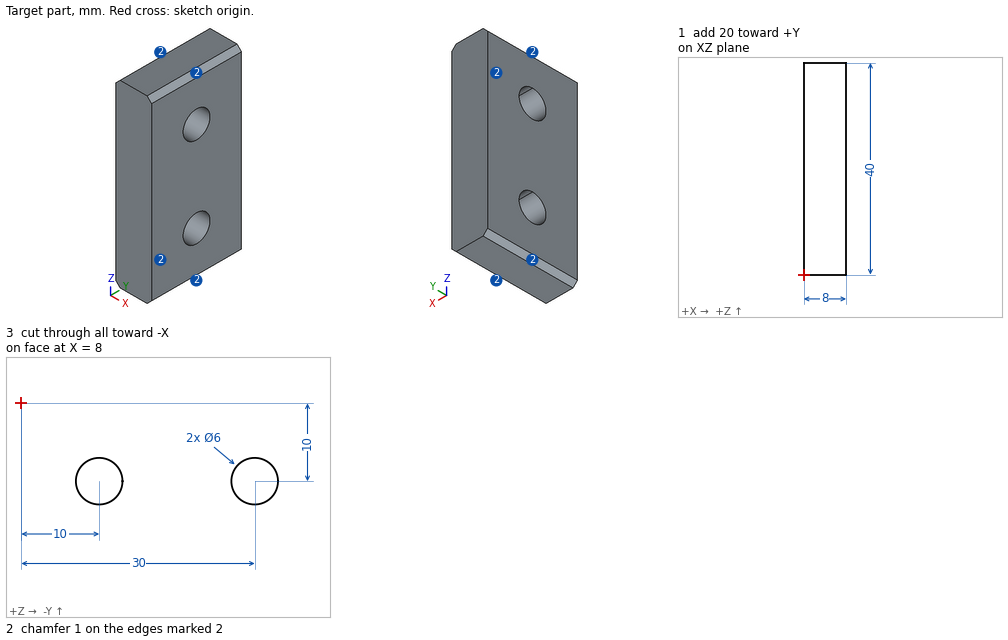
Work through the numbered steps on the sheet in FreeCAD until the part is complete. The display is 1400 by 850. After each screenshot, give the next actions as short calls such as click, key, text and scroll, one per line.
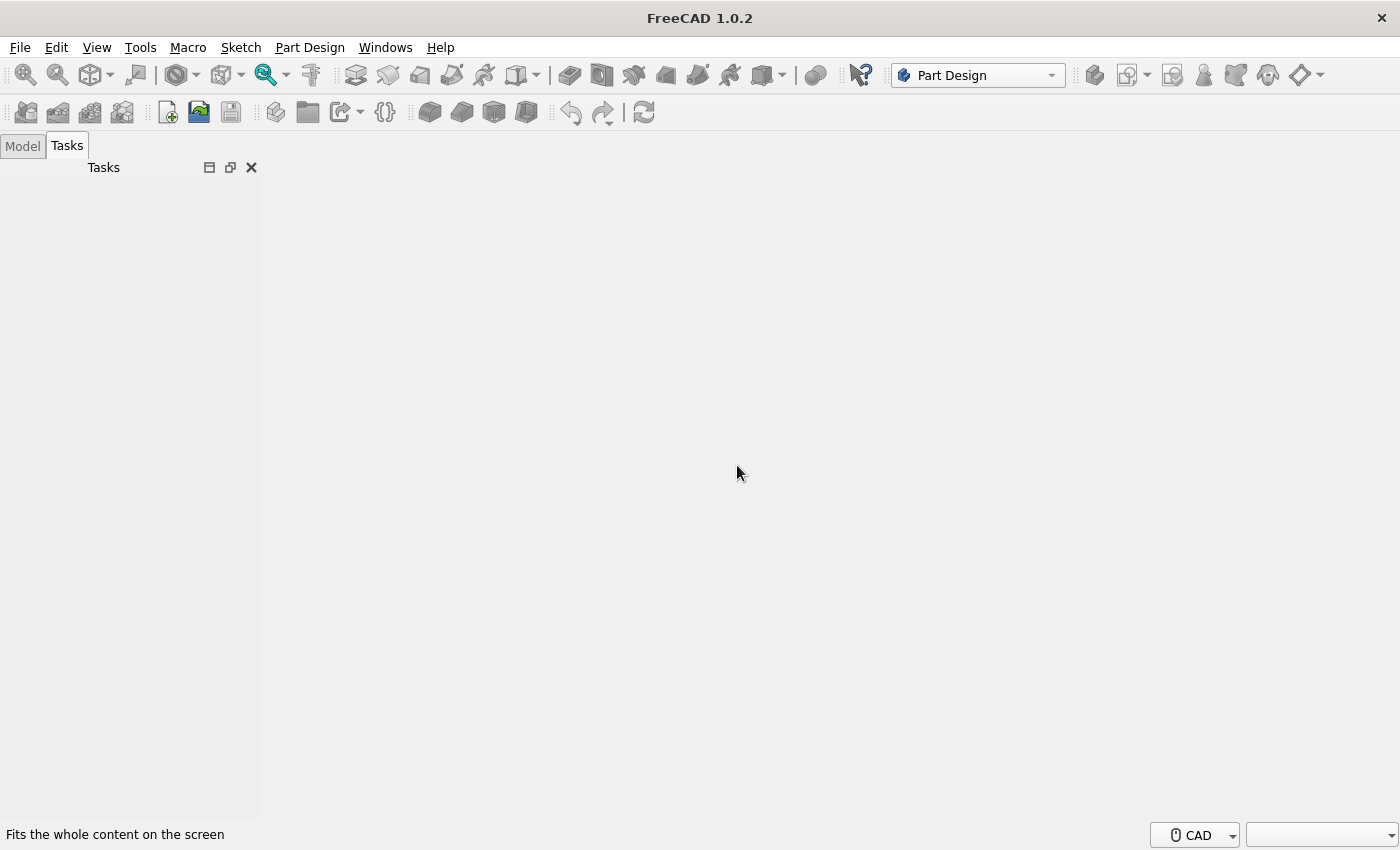
click(168, 112)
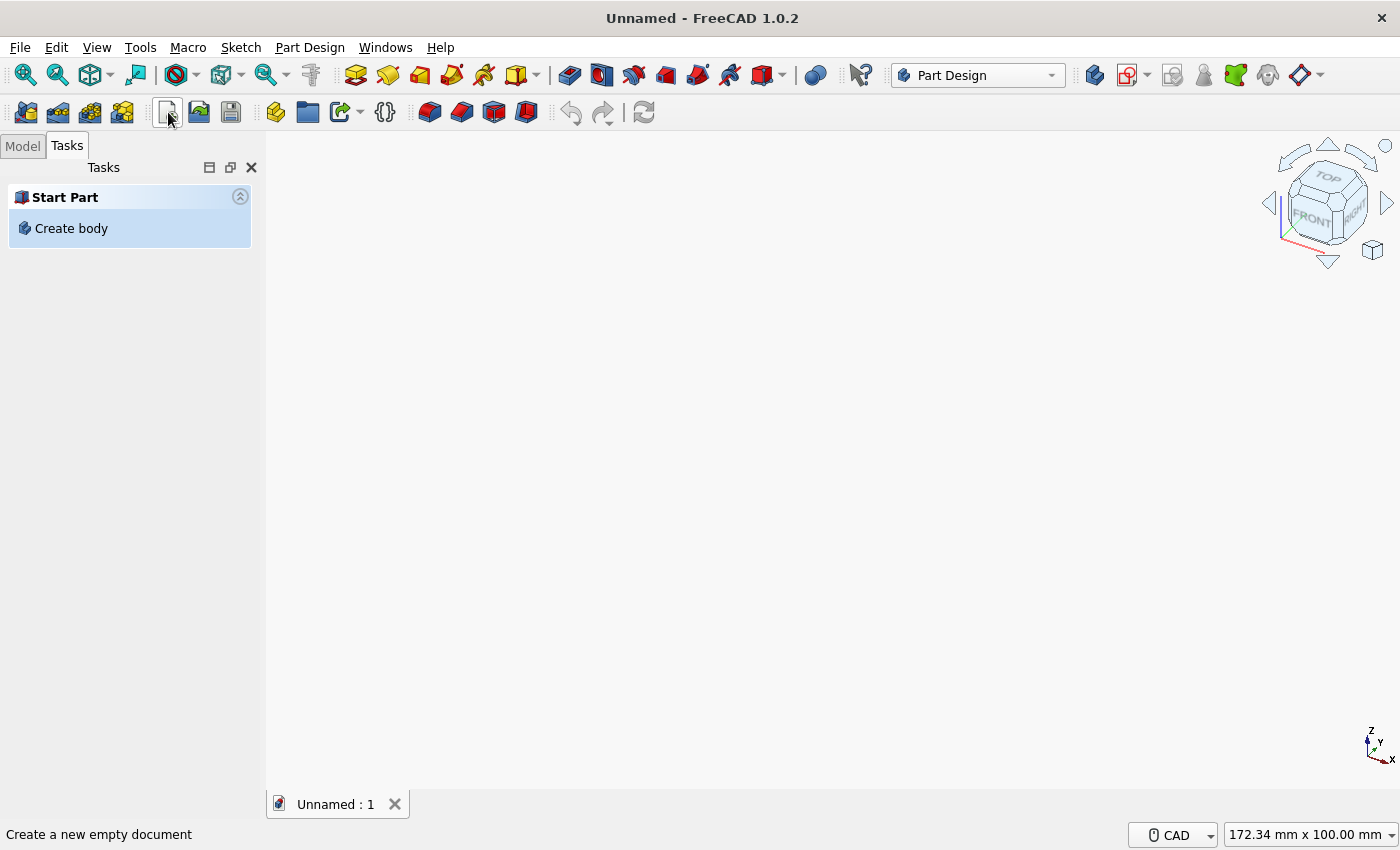
click(1128, 76)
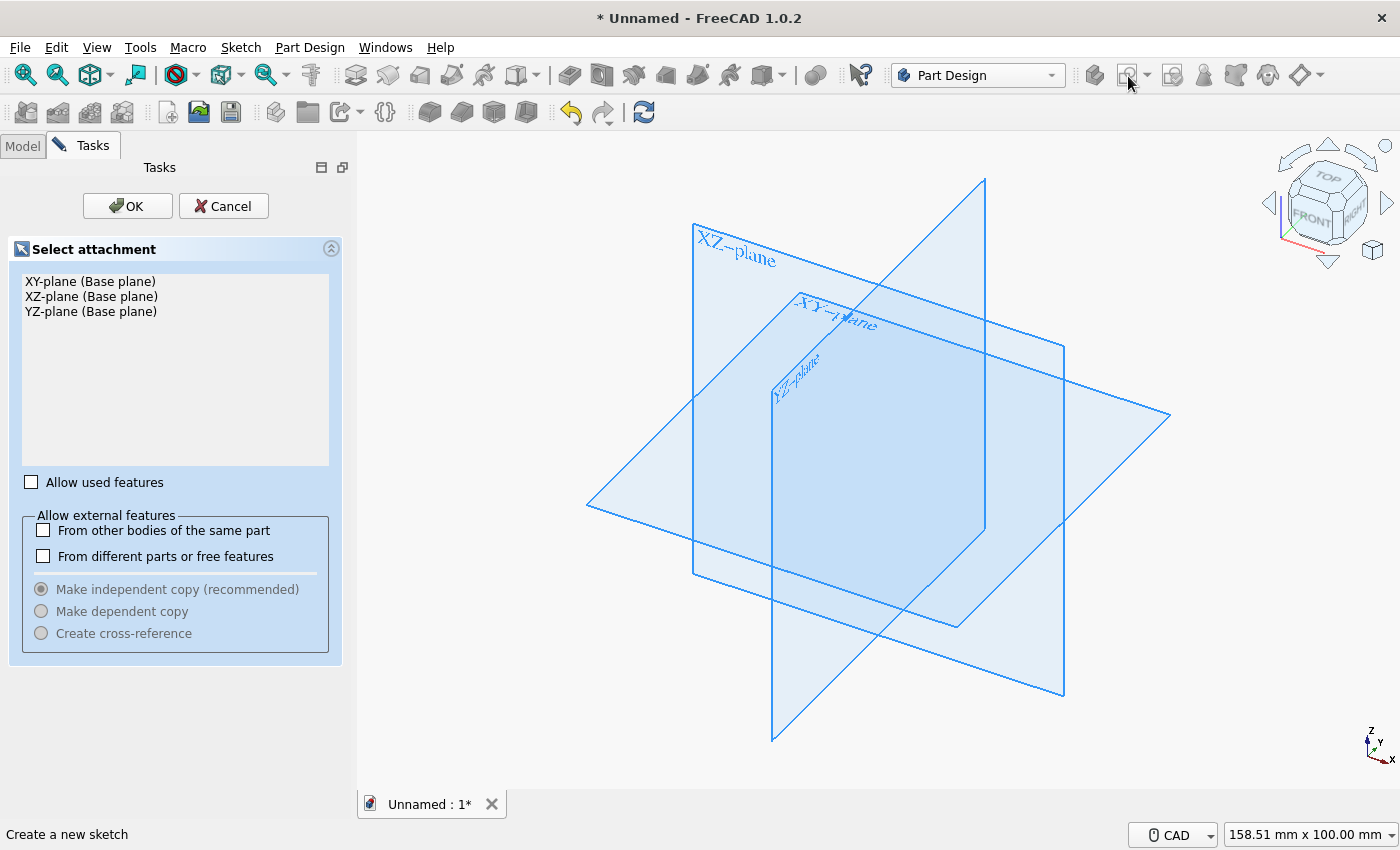
click(82, 296)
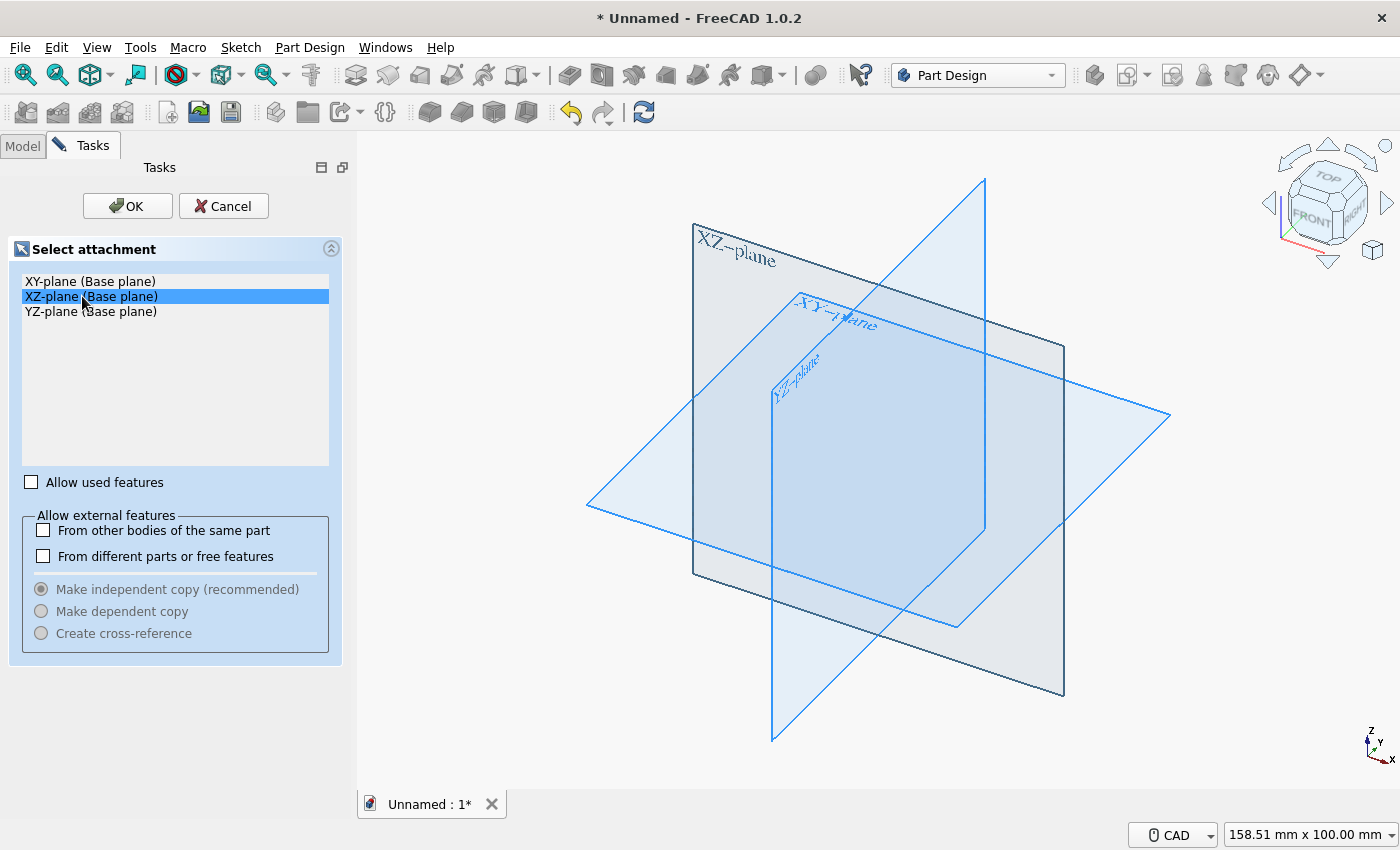
click(128, 206)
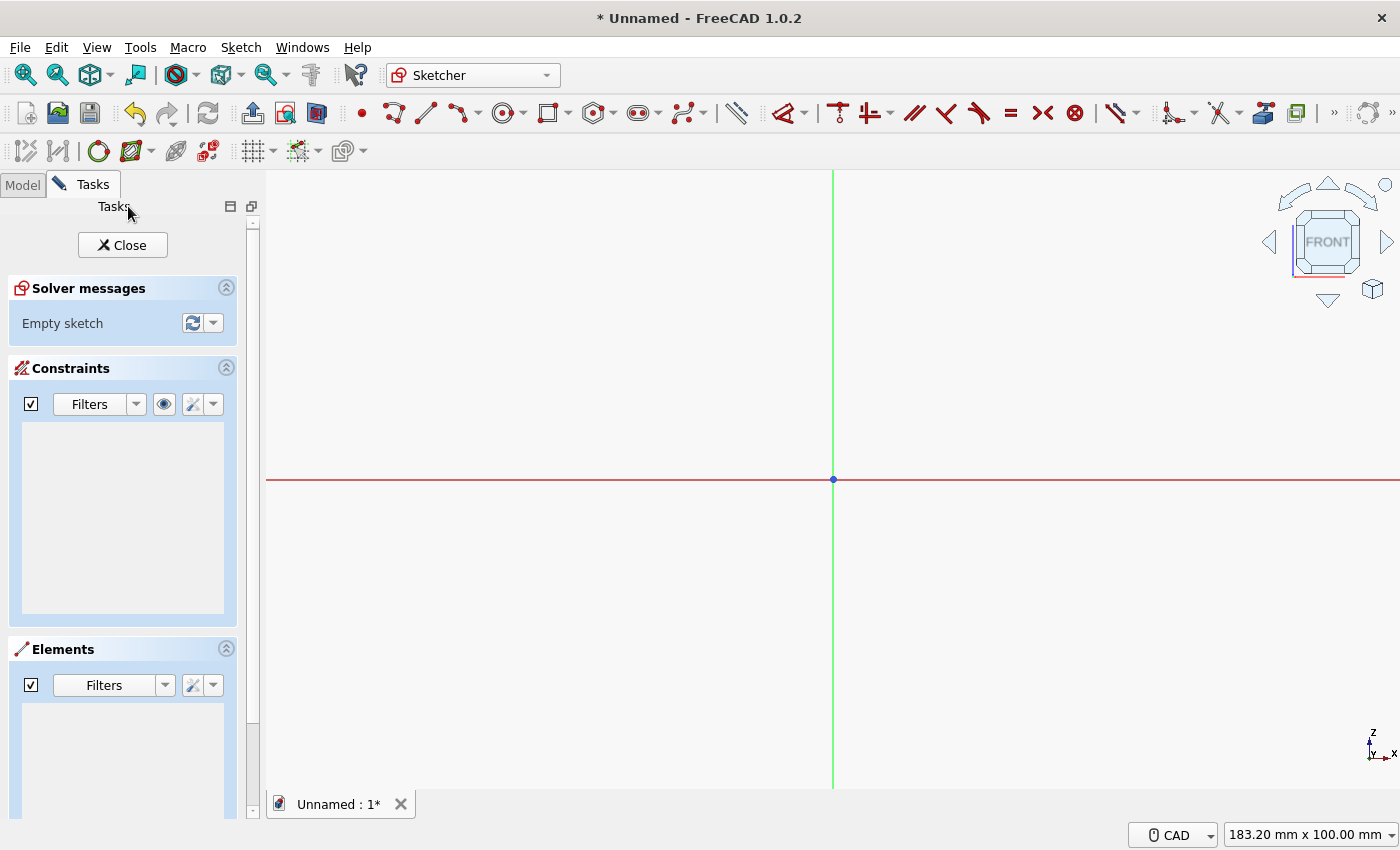
scroll(1047, 198, up, 2)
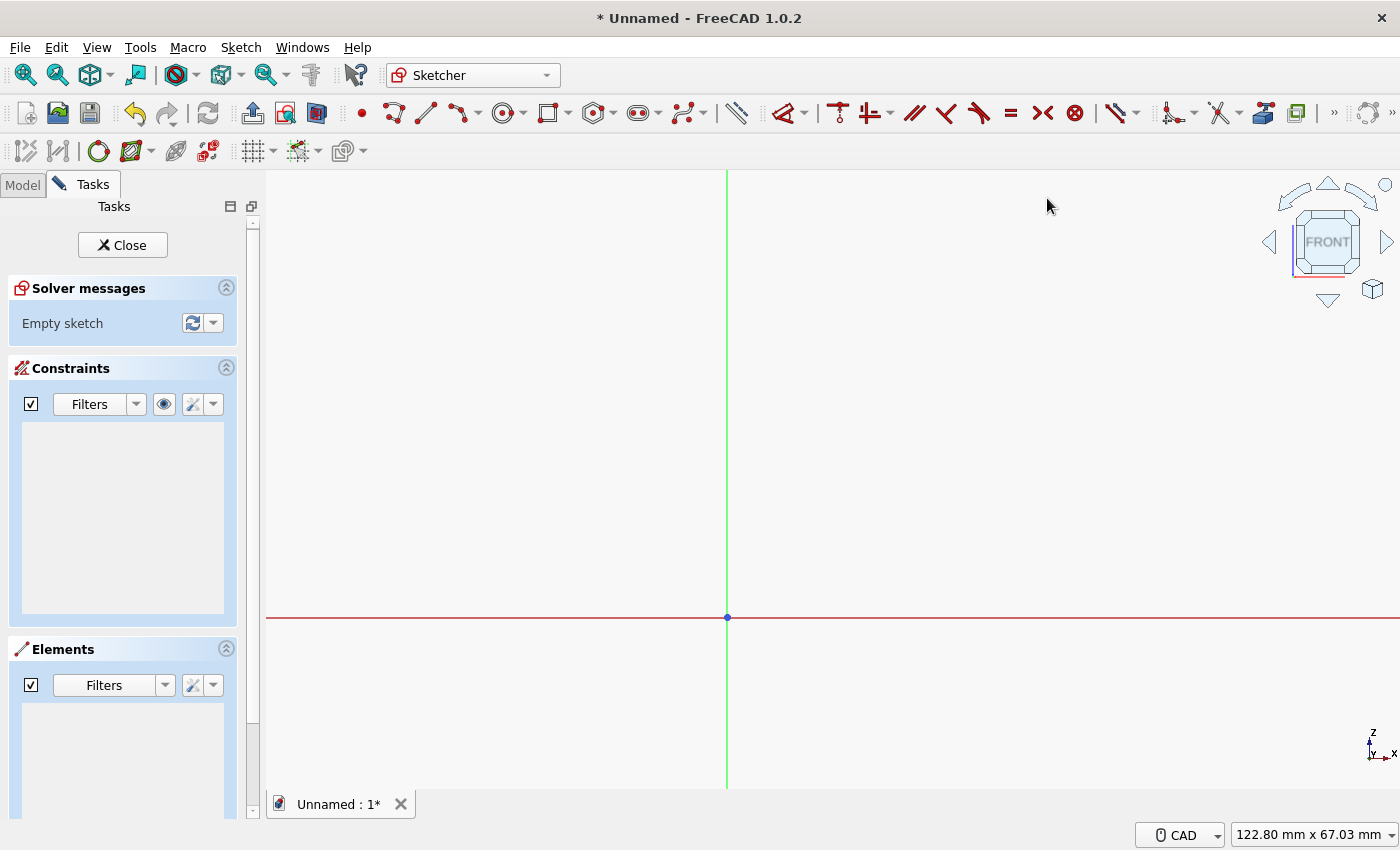
click(548, 114)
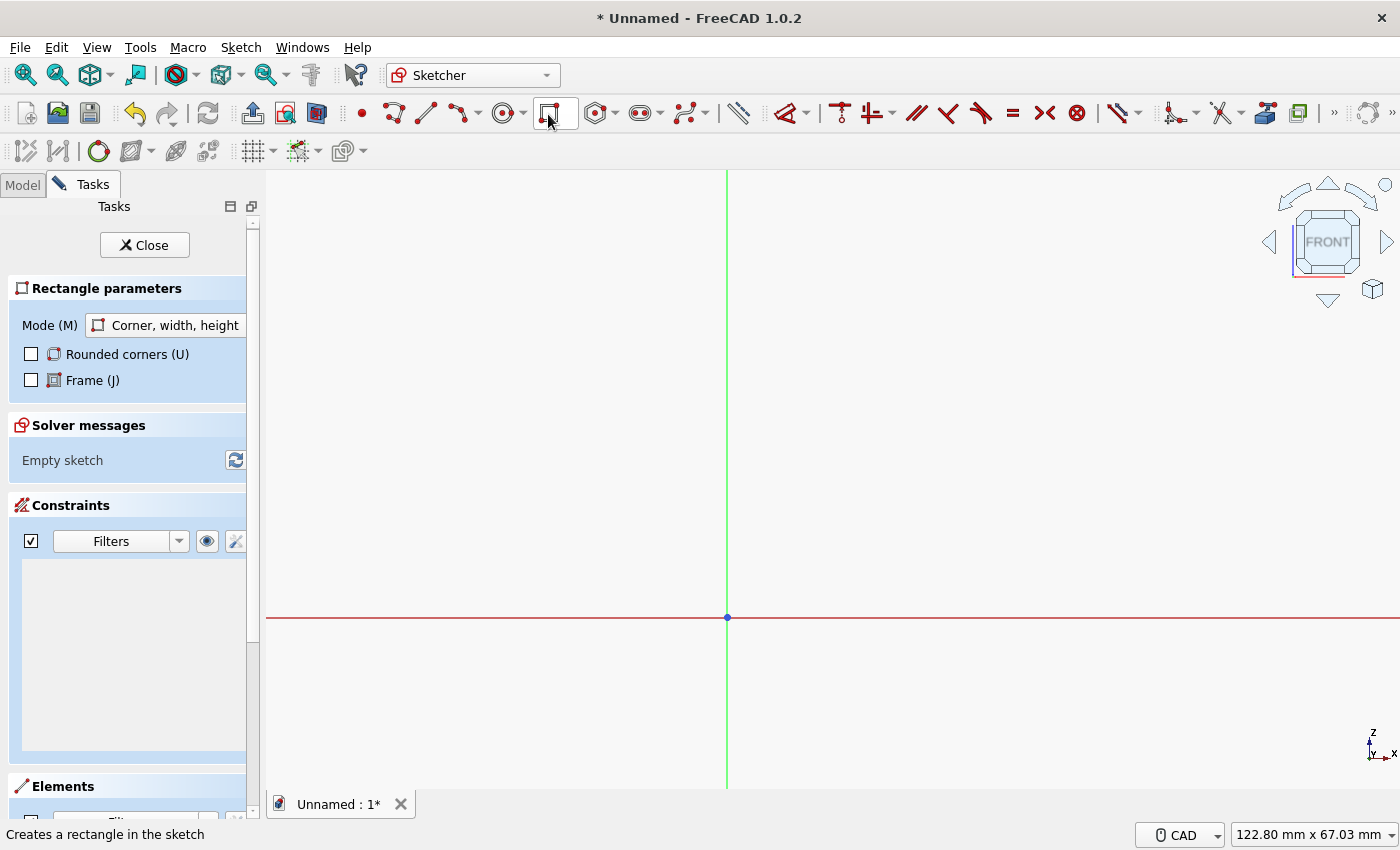
click(727, 618)
move(801, 249)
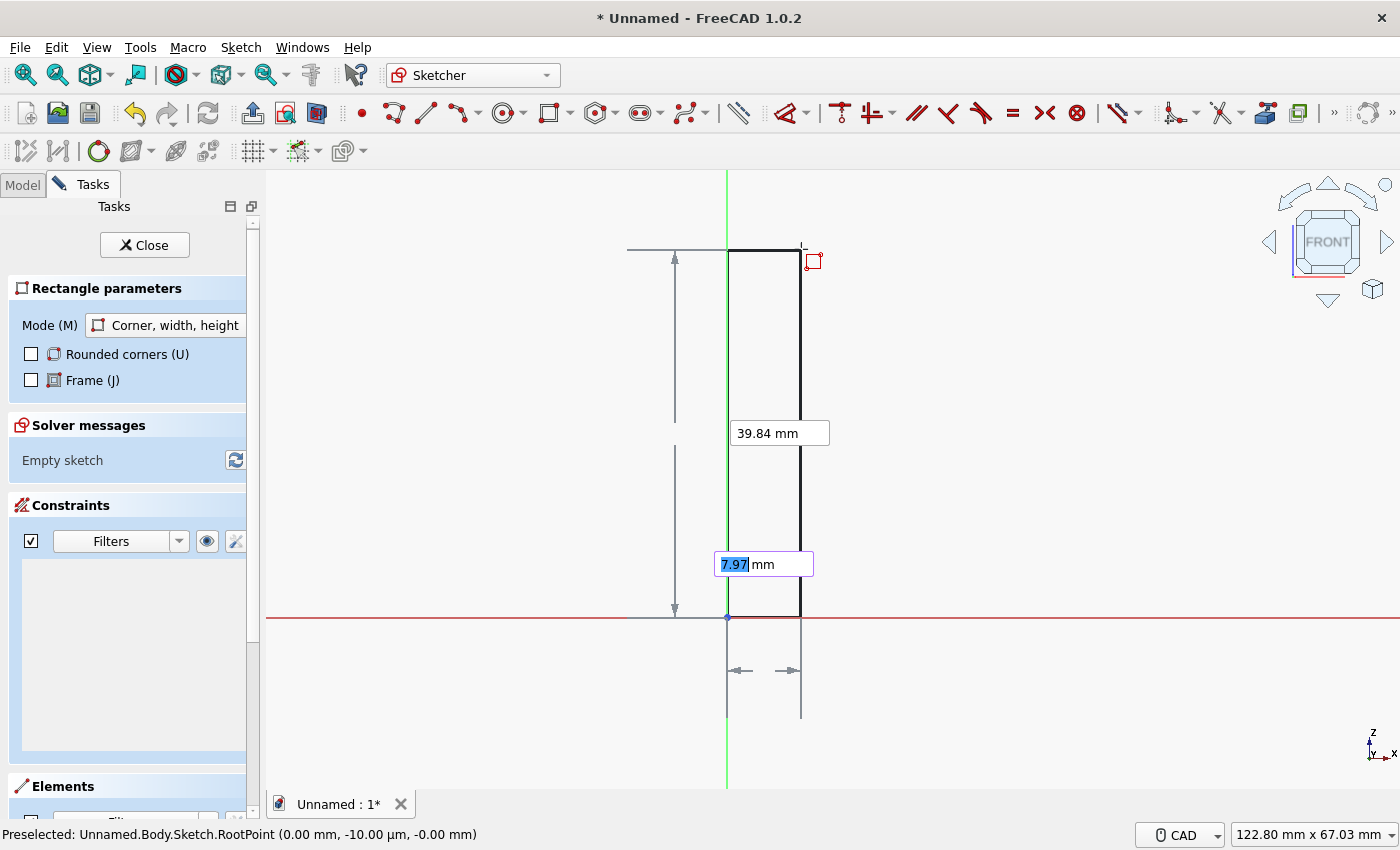
text(8)
key(Tab)
text(40)
key(Return)
key(Escape)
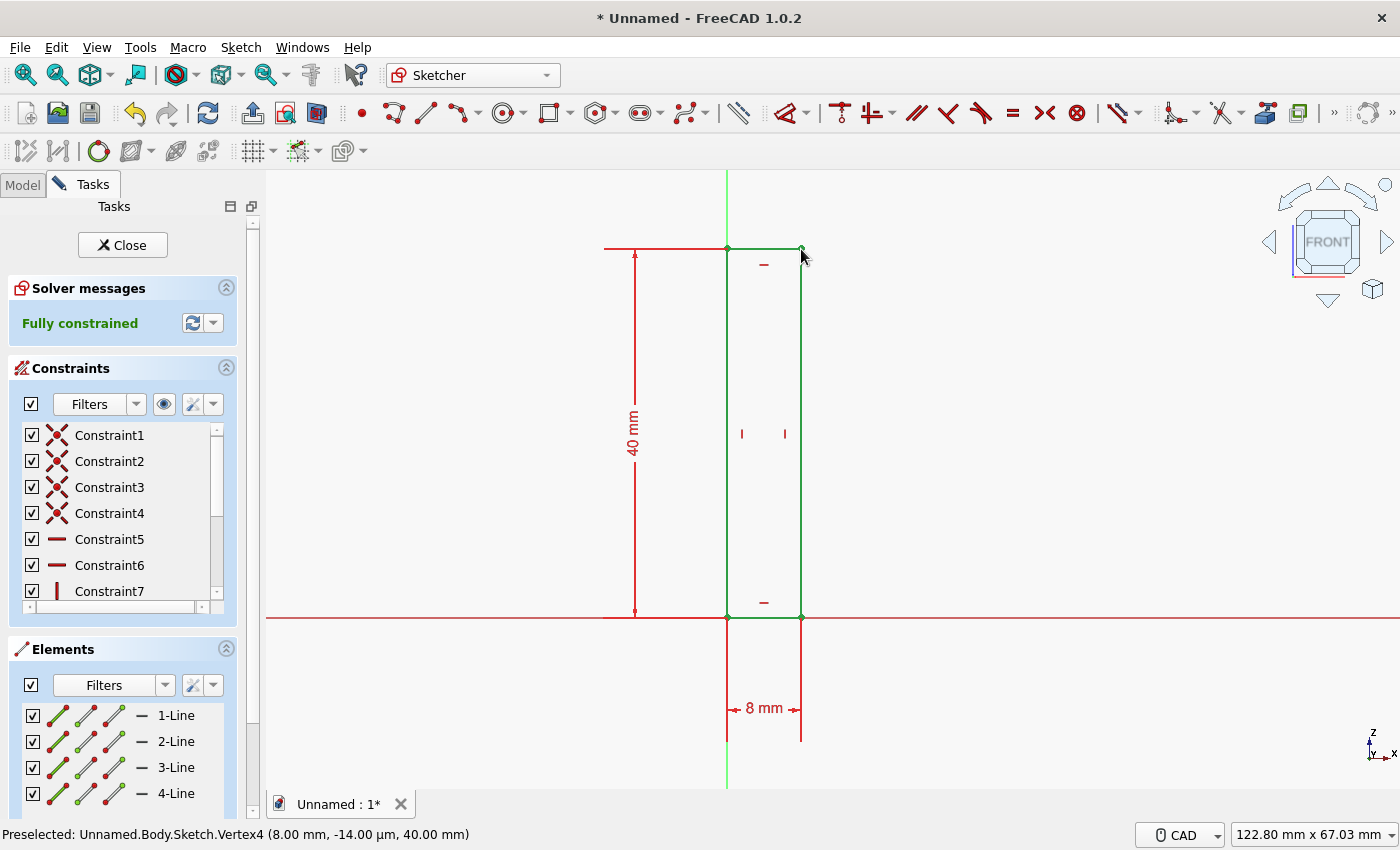
click(123, 245)